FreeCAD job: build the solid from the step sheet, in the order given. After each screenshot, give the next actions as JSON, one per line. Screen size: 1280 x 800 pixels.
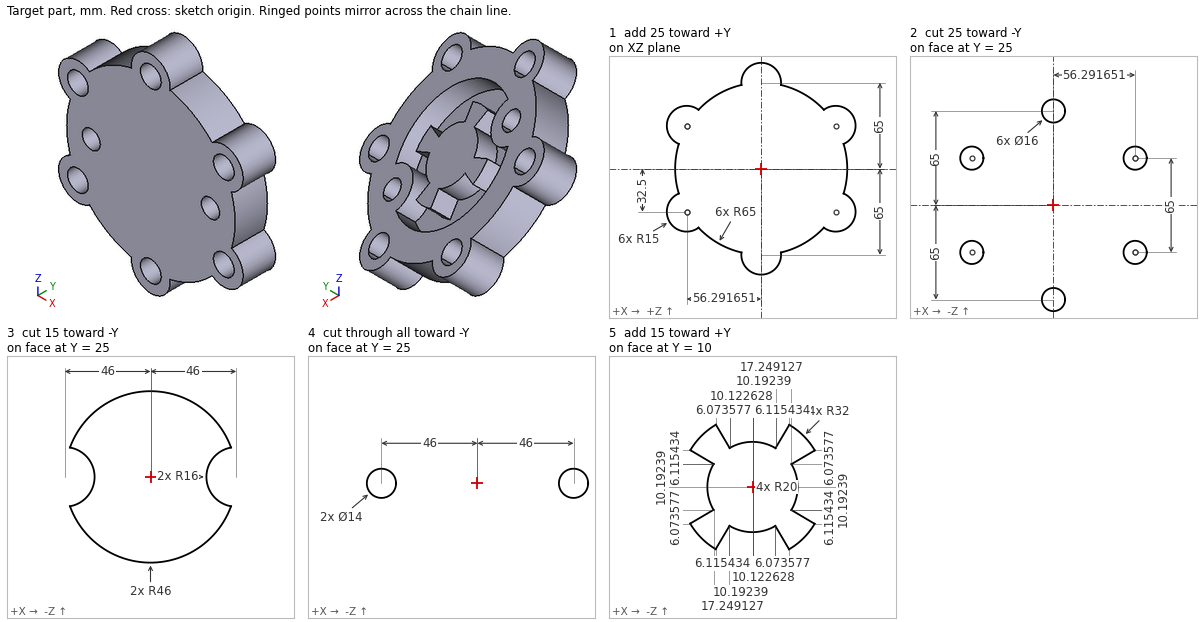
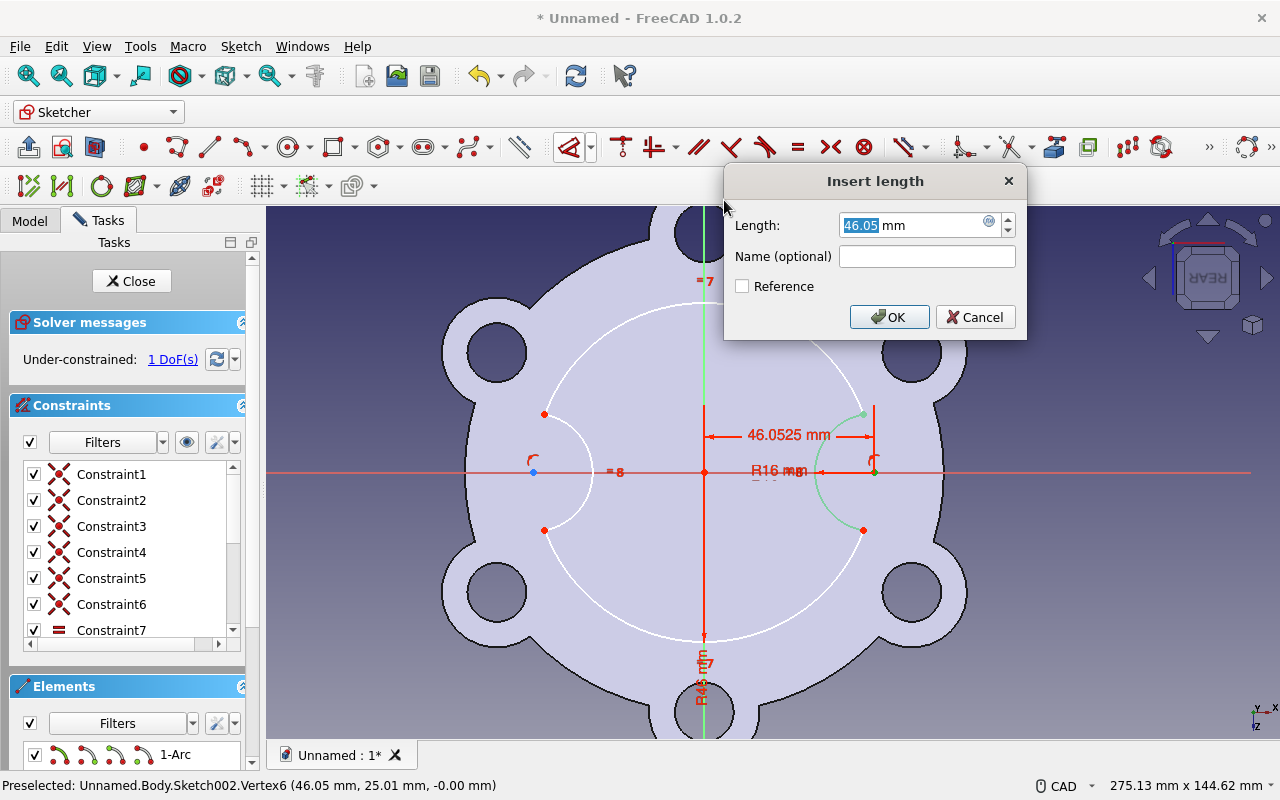
{"action": "type", "text": "46"}
{"action": "key", "text": "Return"}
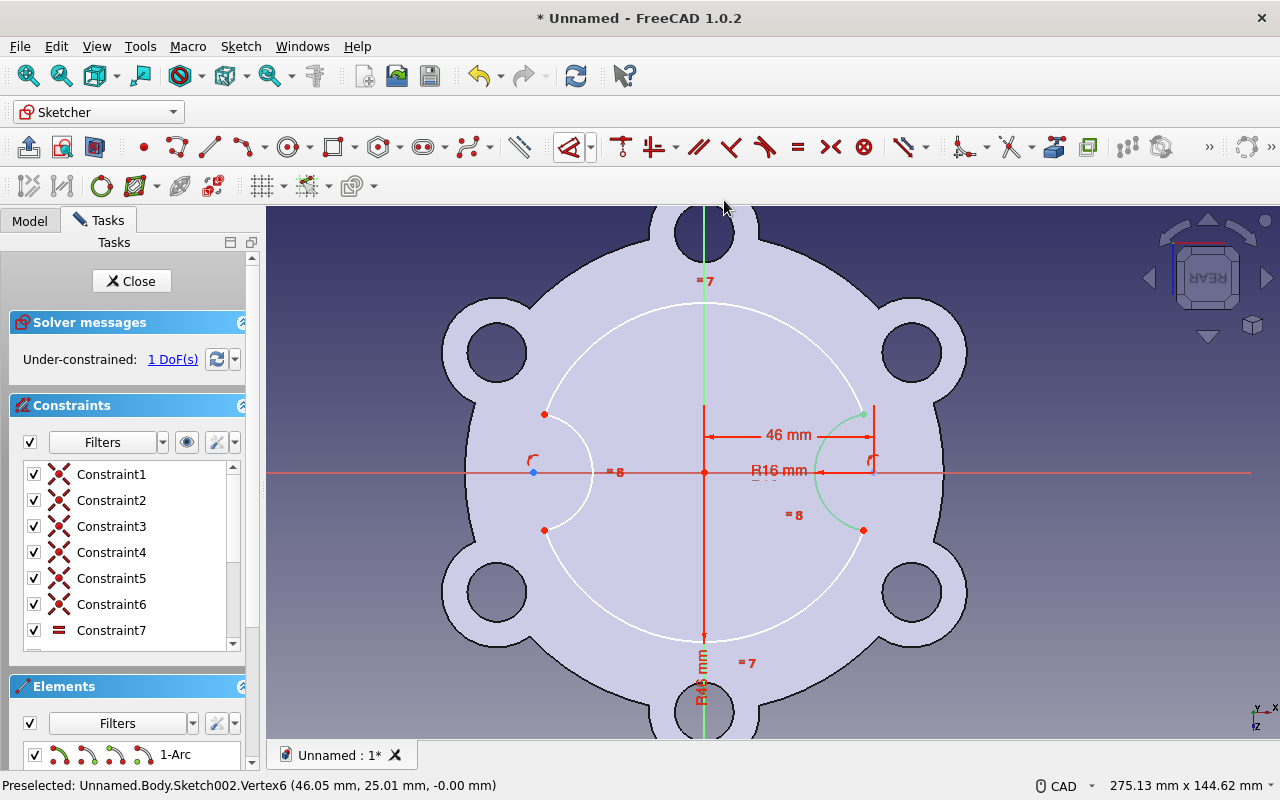
{"action": "left_click", "coordinate": [534, 472]}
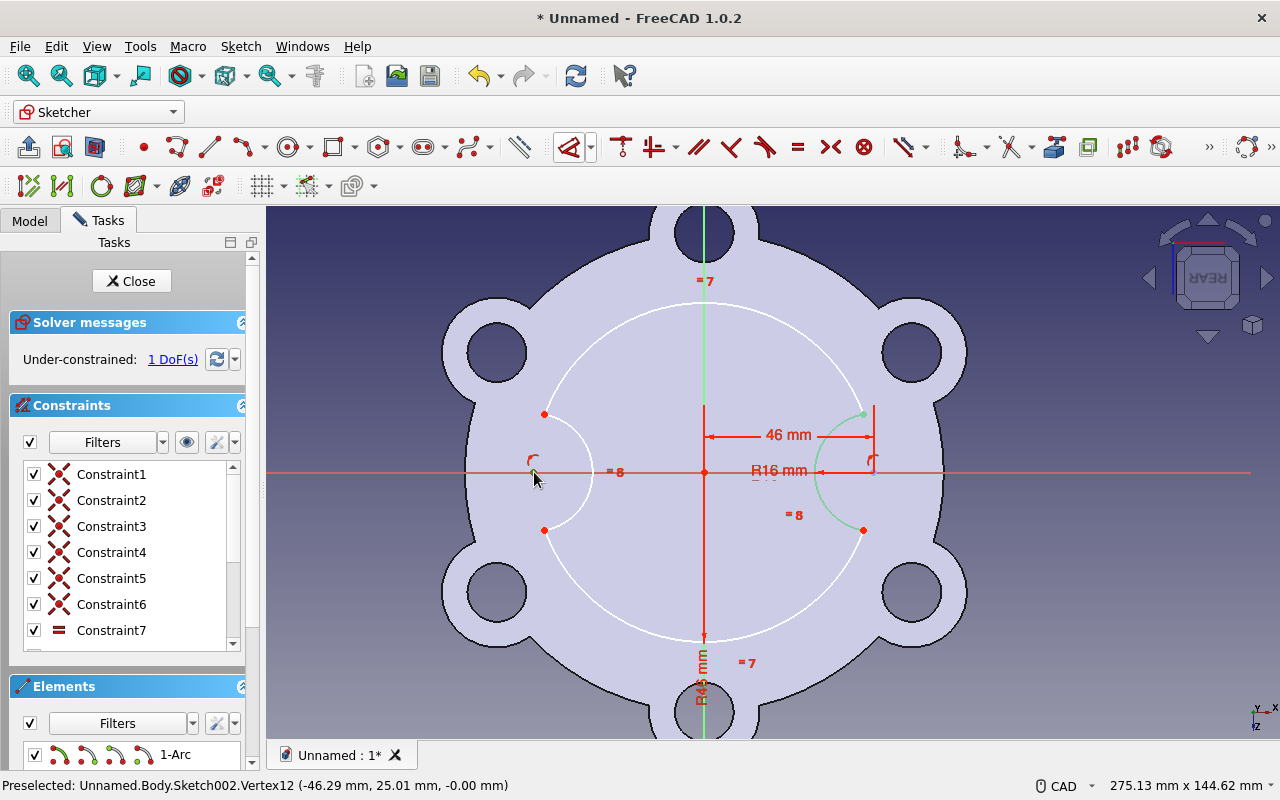
{"action": "key", "text": "l"}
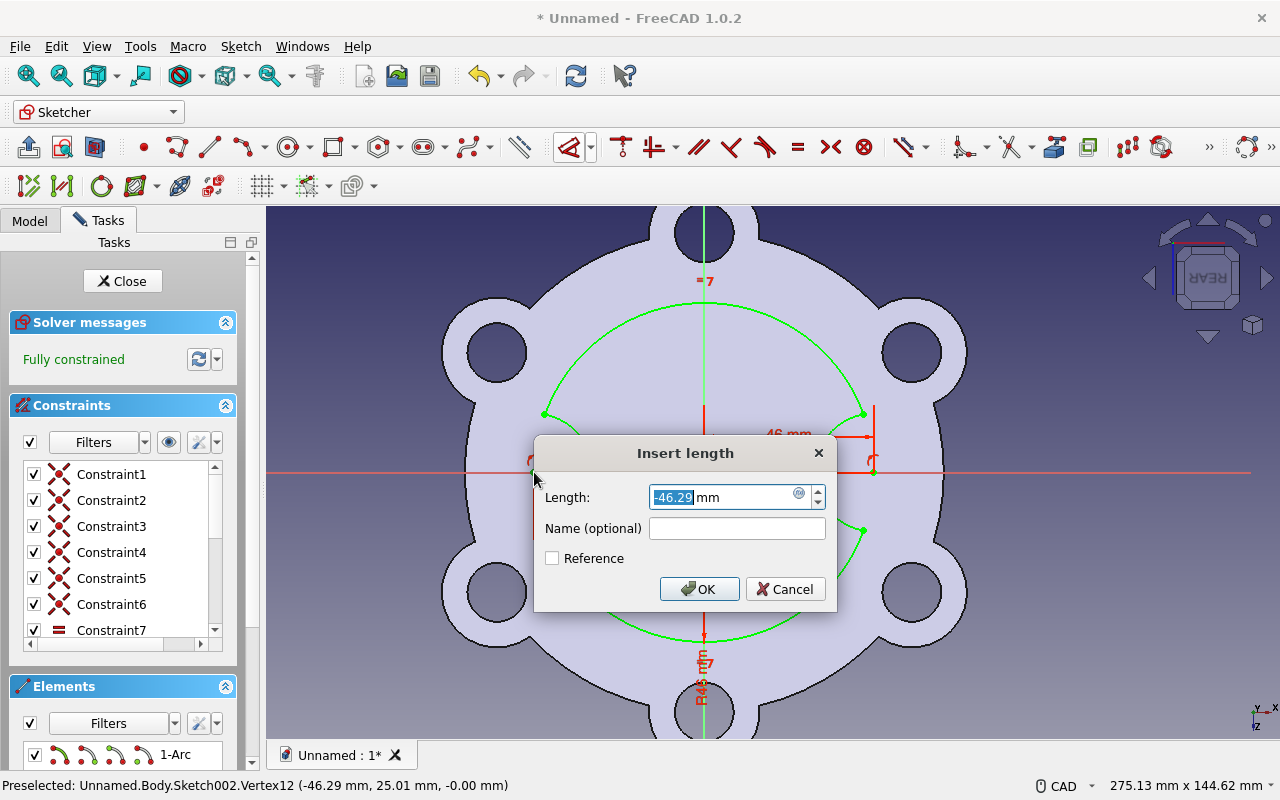
{"action": "type", "text": "-46"}
{"action": "key", "text": "Return"}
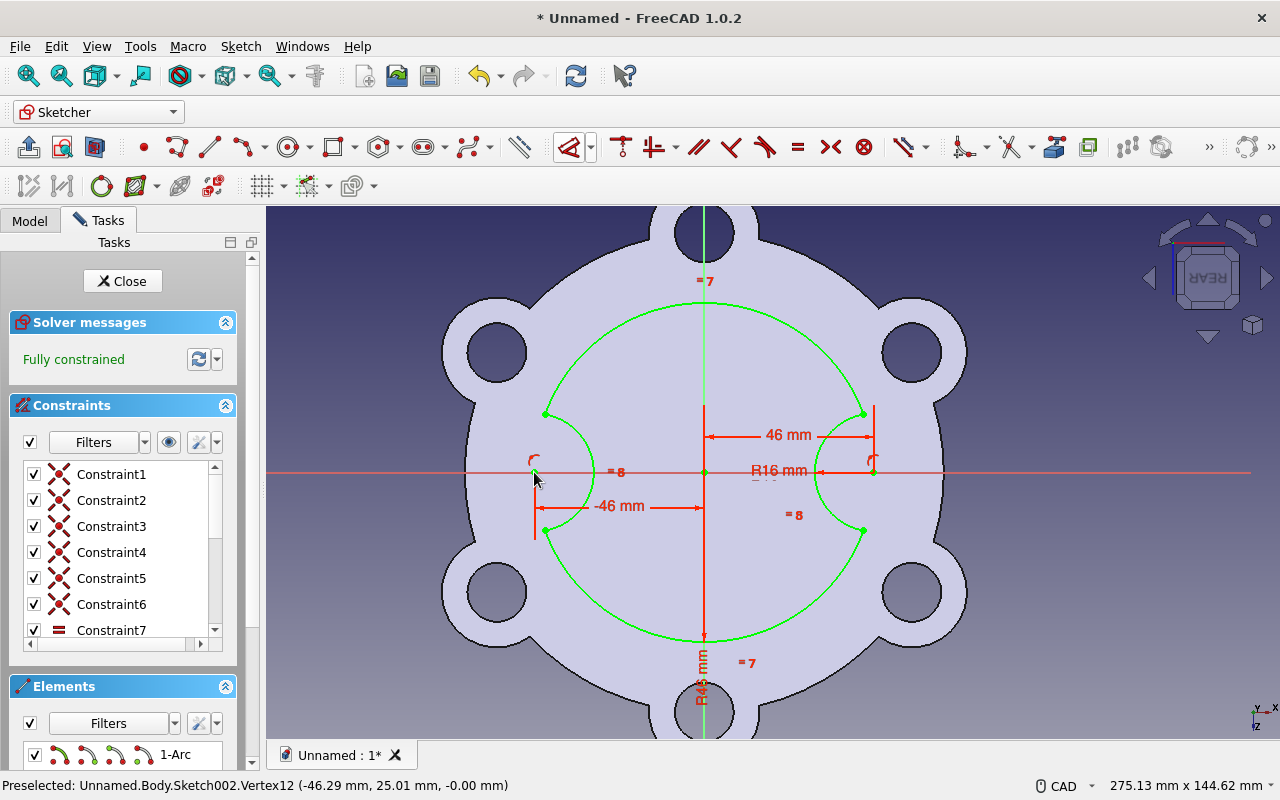
{"action": "left_click", "coordinate": [123, 281]}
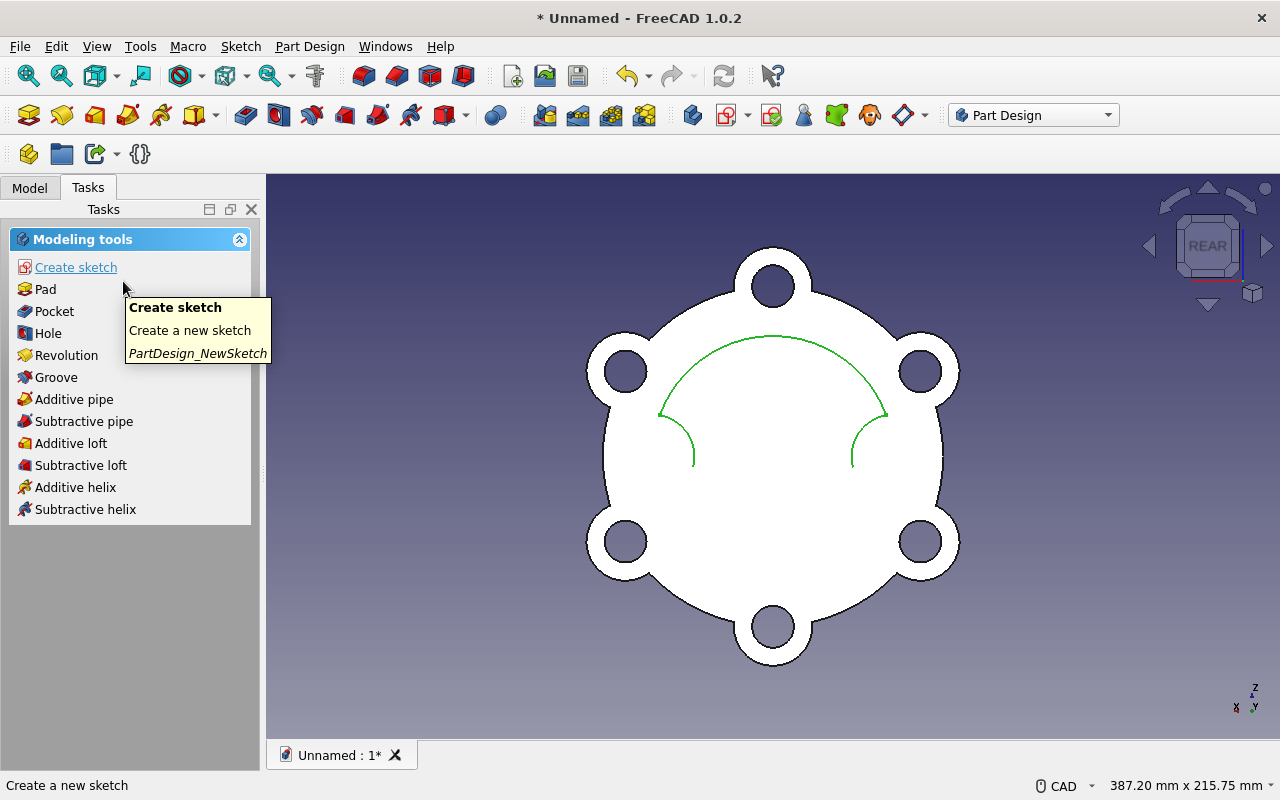
{"action": "left_click", "coordinate": [246, 116]}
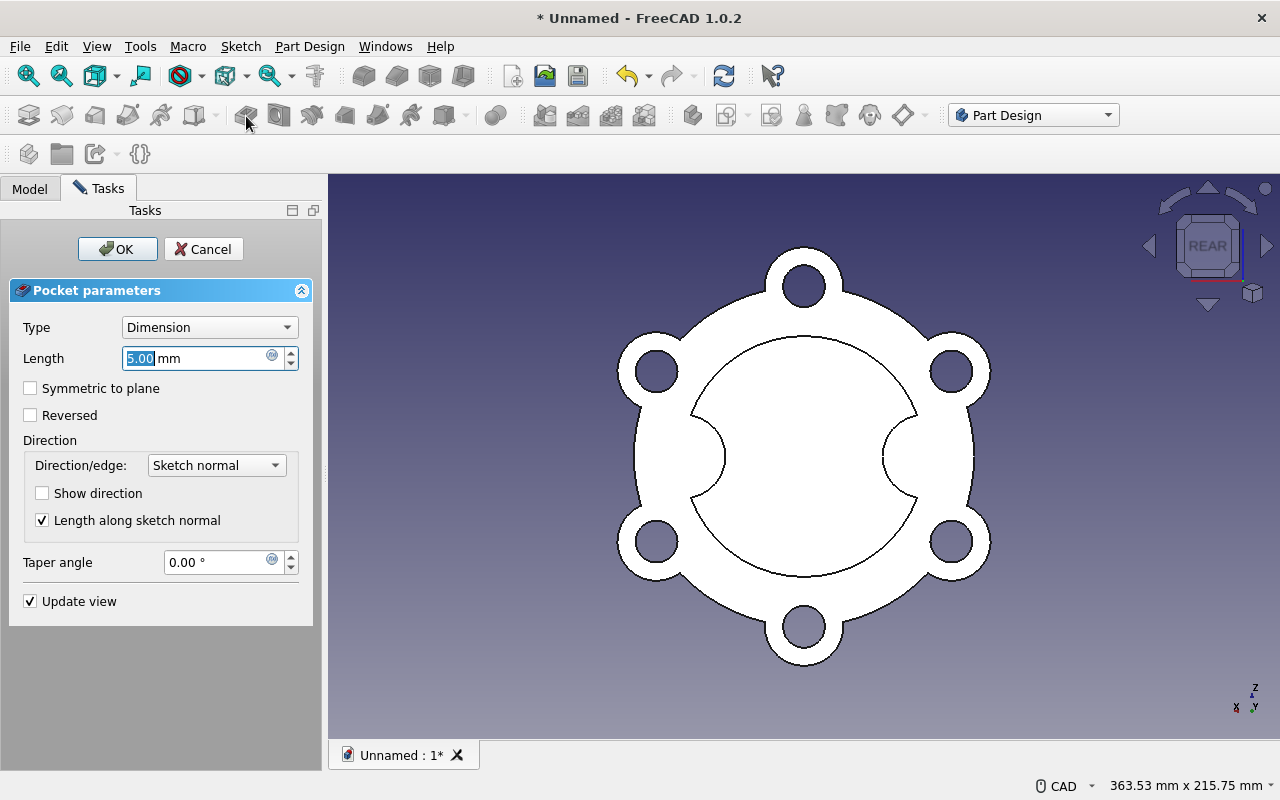
{"action": "type", "text": "15"}
{"action": "key", "text": "Tab"}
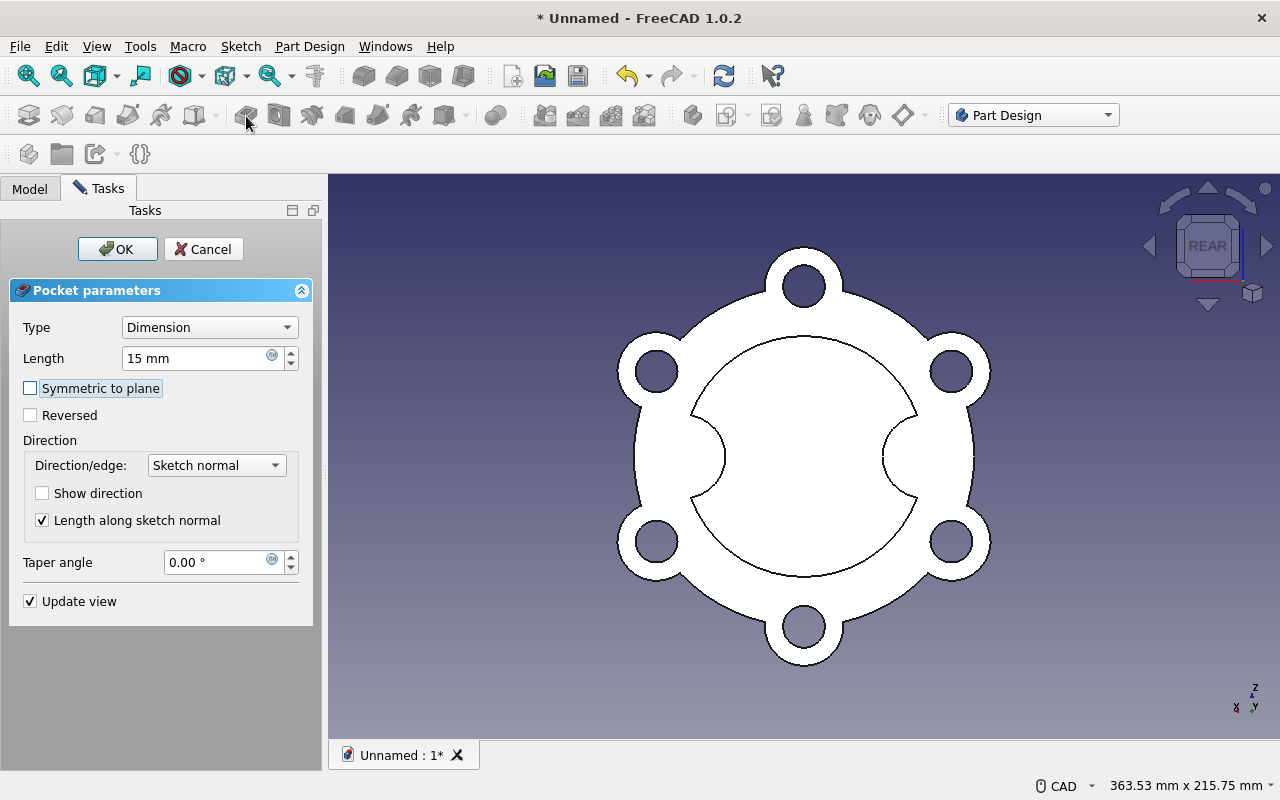
{"action": "left_click", "coordinate": [118, 249]}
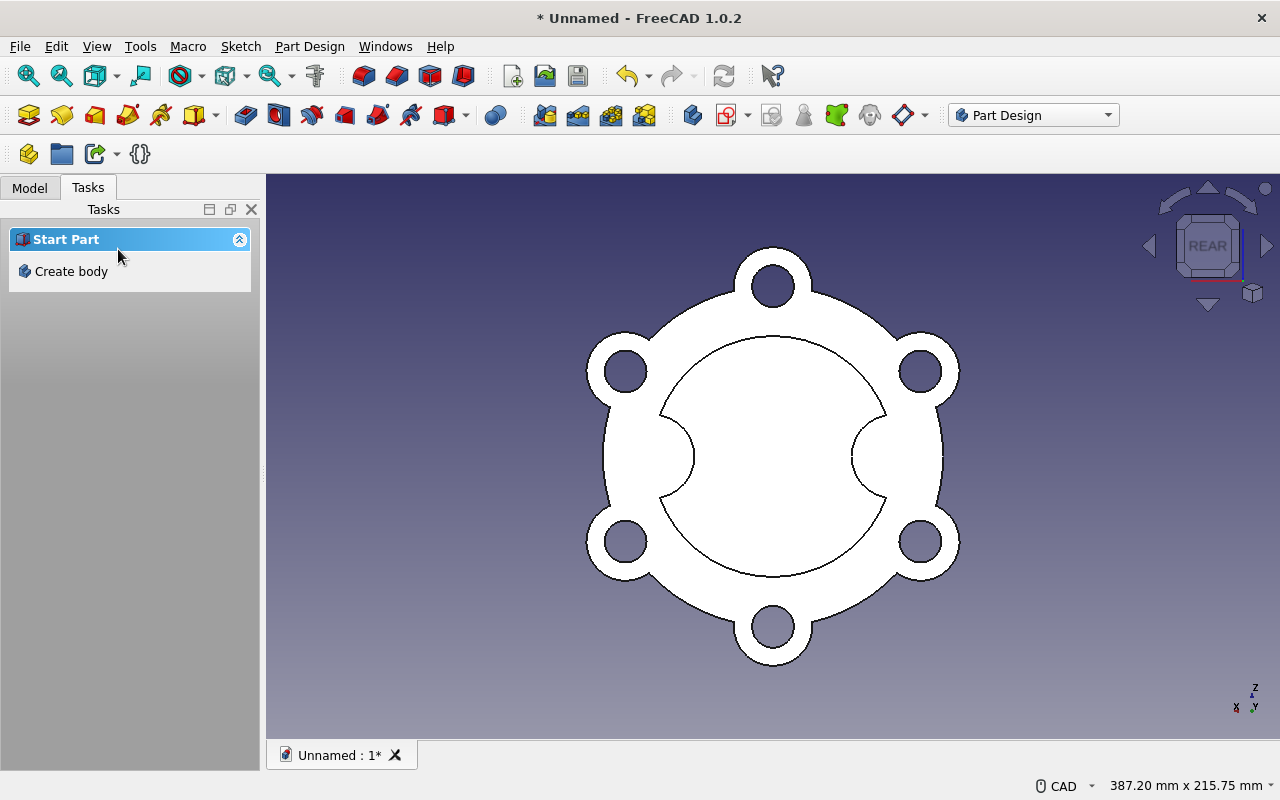
{"action": "left_click", "coordinate": [666, 455]}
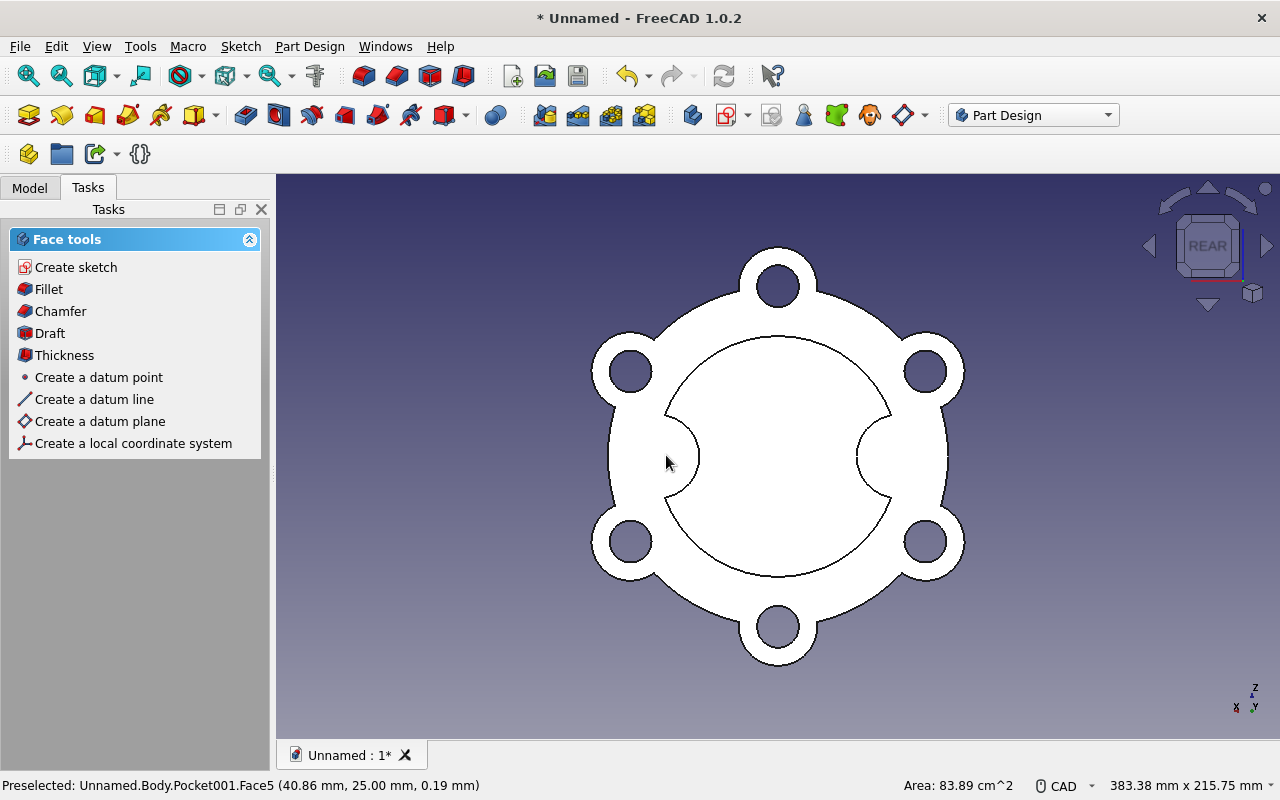
{"action": "left_click", "coordinate": [726, 116]}